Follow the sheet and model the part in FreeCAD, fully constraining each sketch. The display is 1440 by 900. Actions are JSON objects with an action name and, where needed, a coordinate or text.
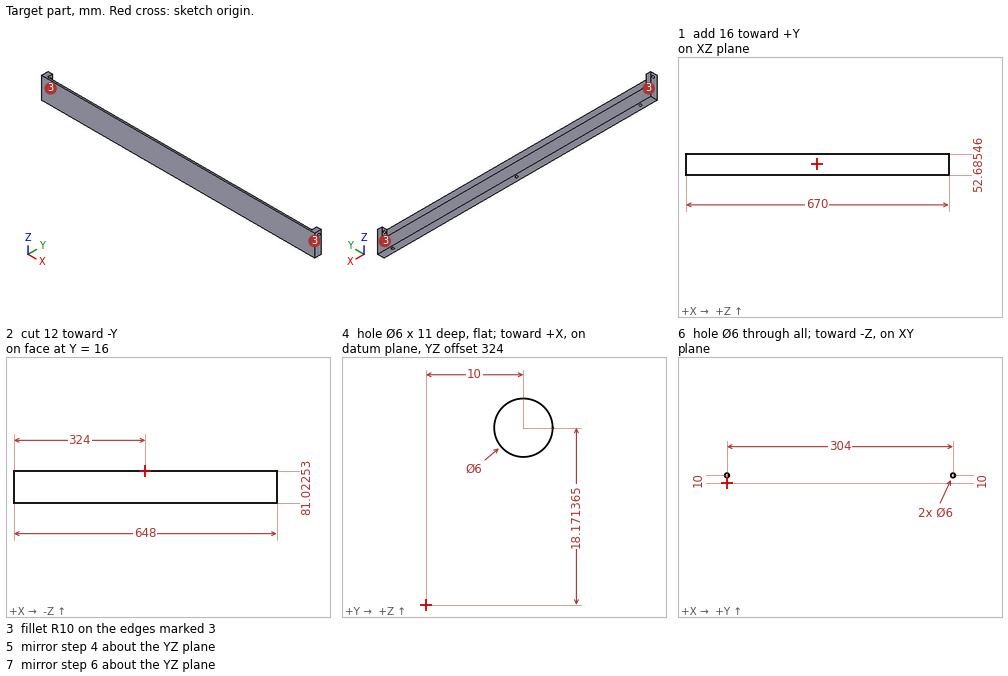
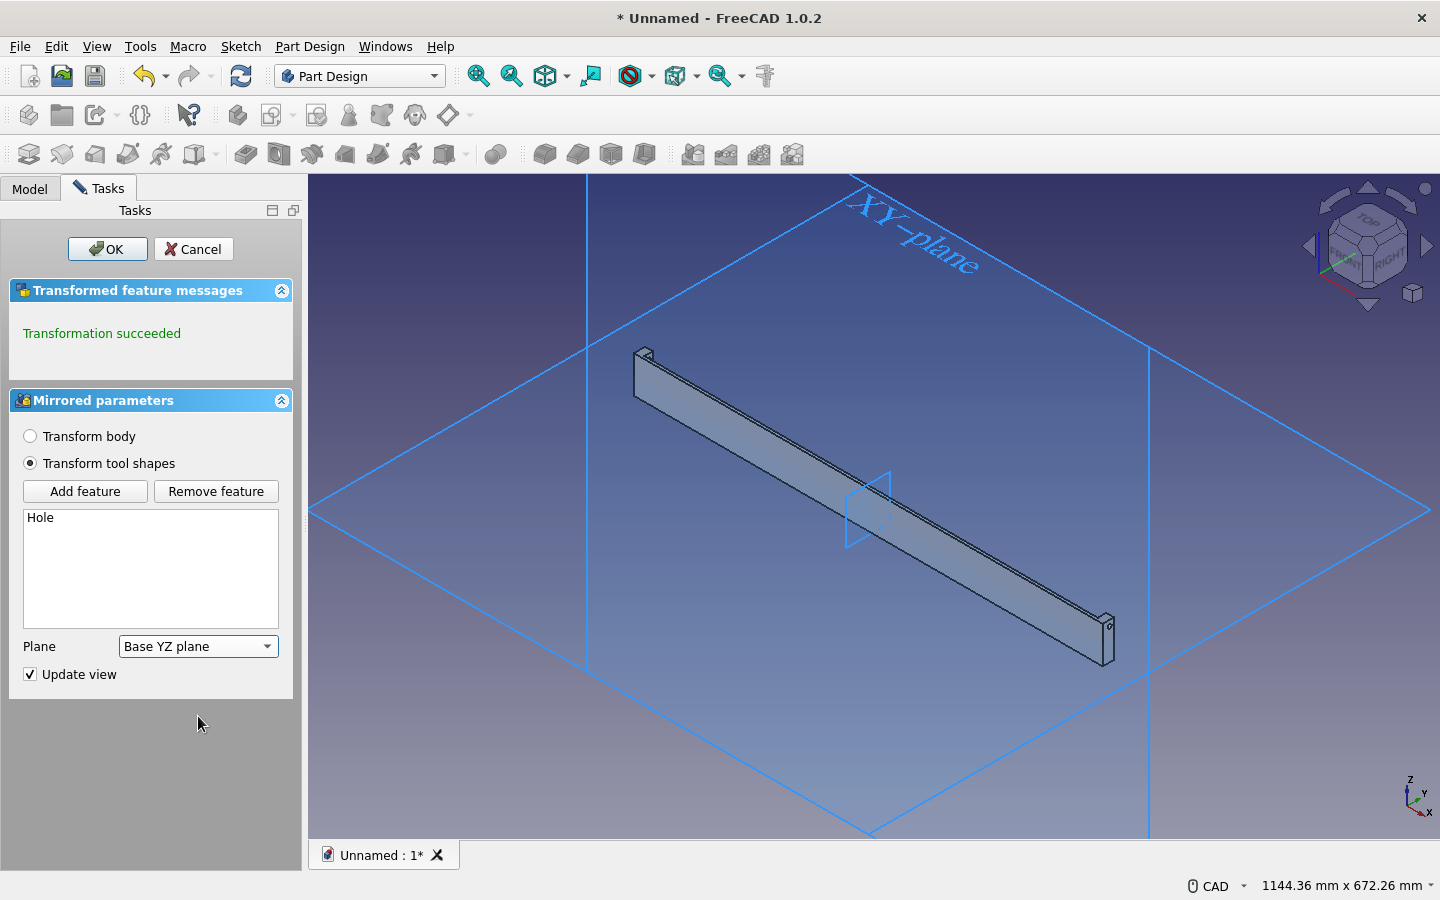
{"action": "left_click", "coordinate": [108, 249]}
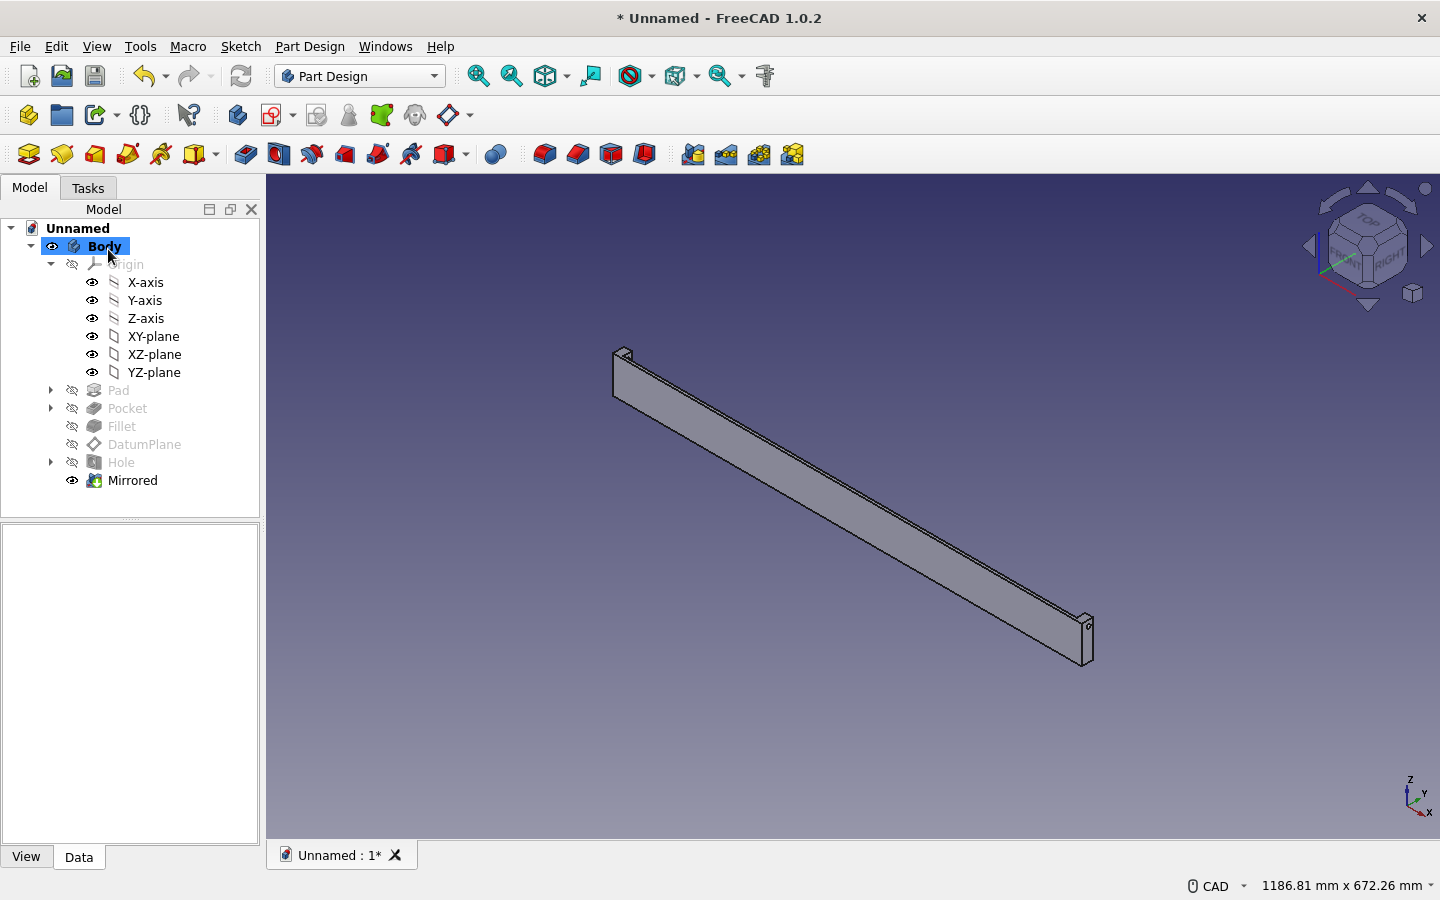
{"action": "left_click", "coordinate": [270, 116]}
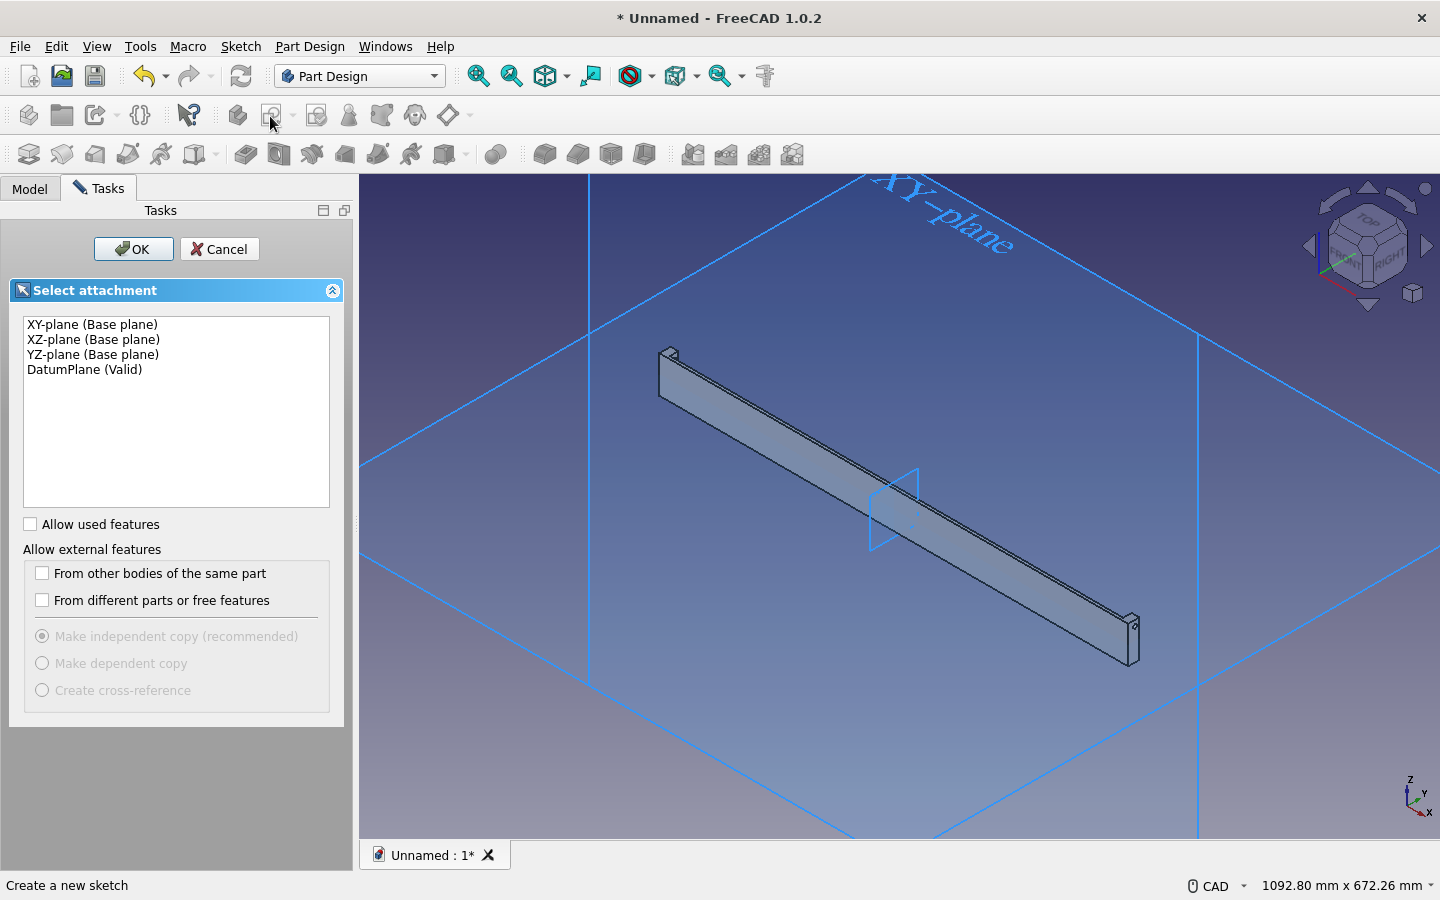
{"action": "left_click", "coordinate": [84, 324]}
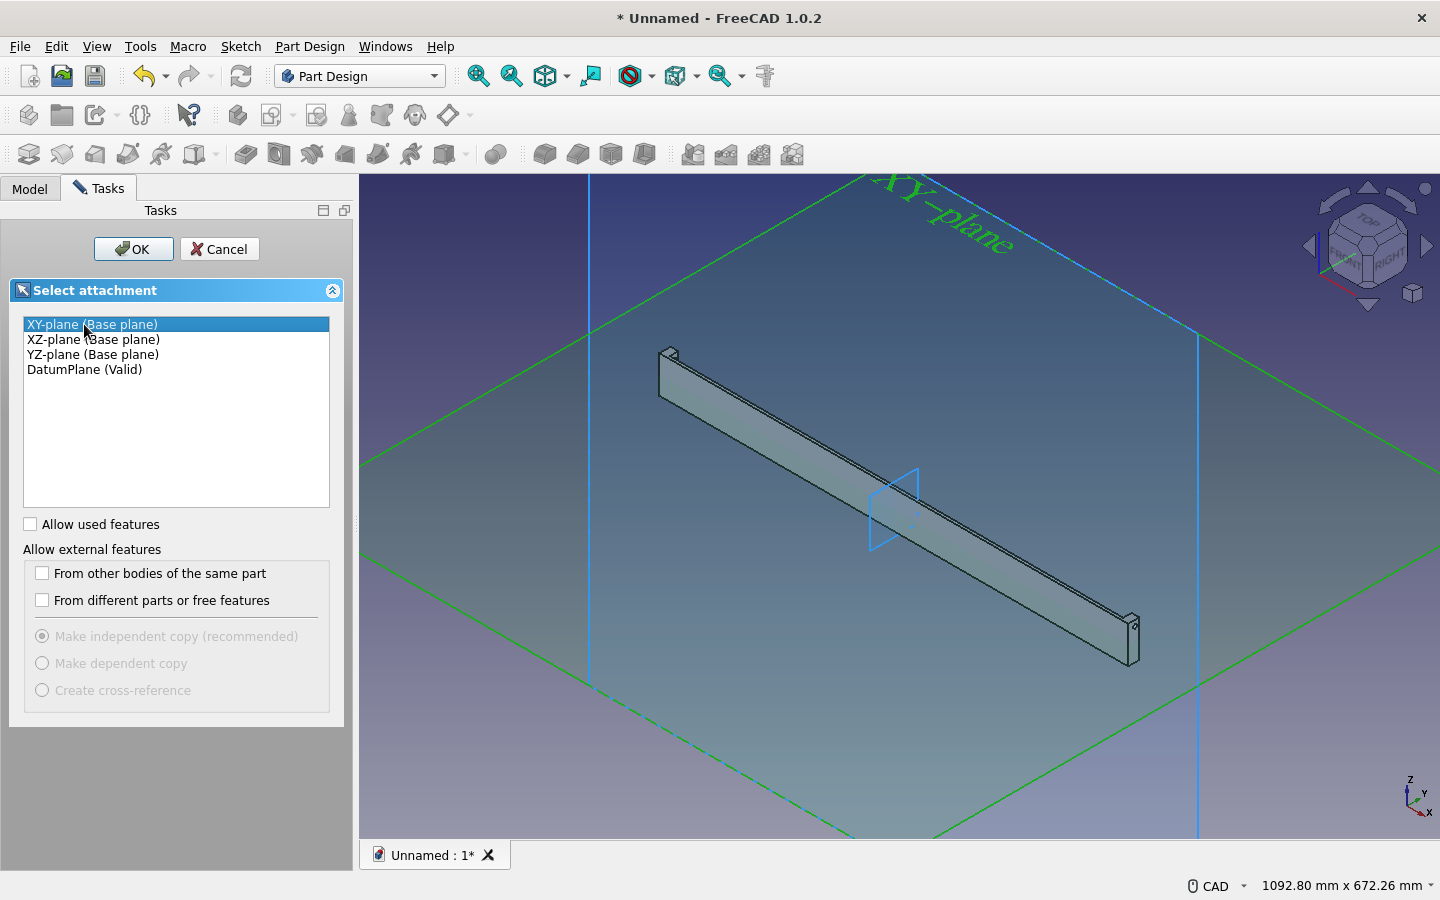
{"action": "left_click", "coordinate": [134, 249]}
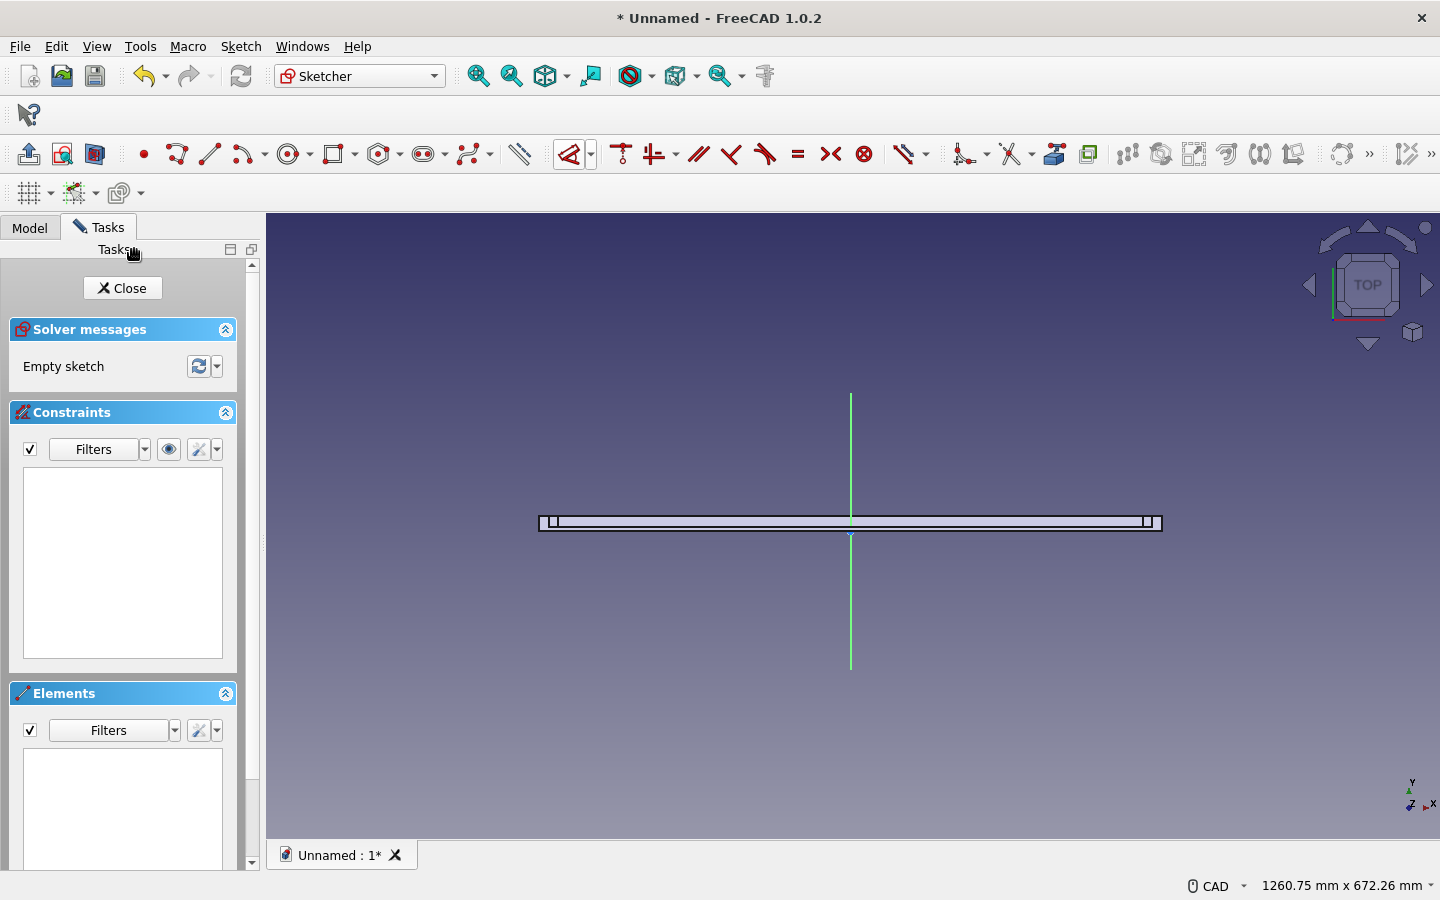
{"action": "left_click", "coordinate": [95, 154]}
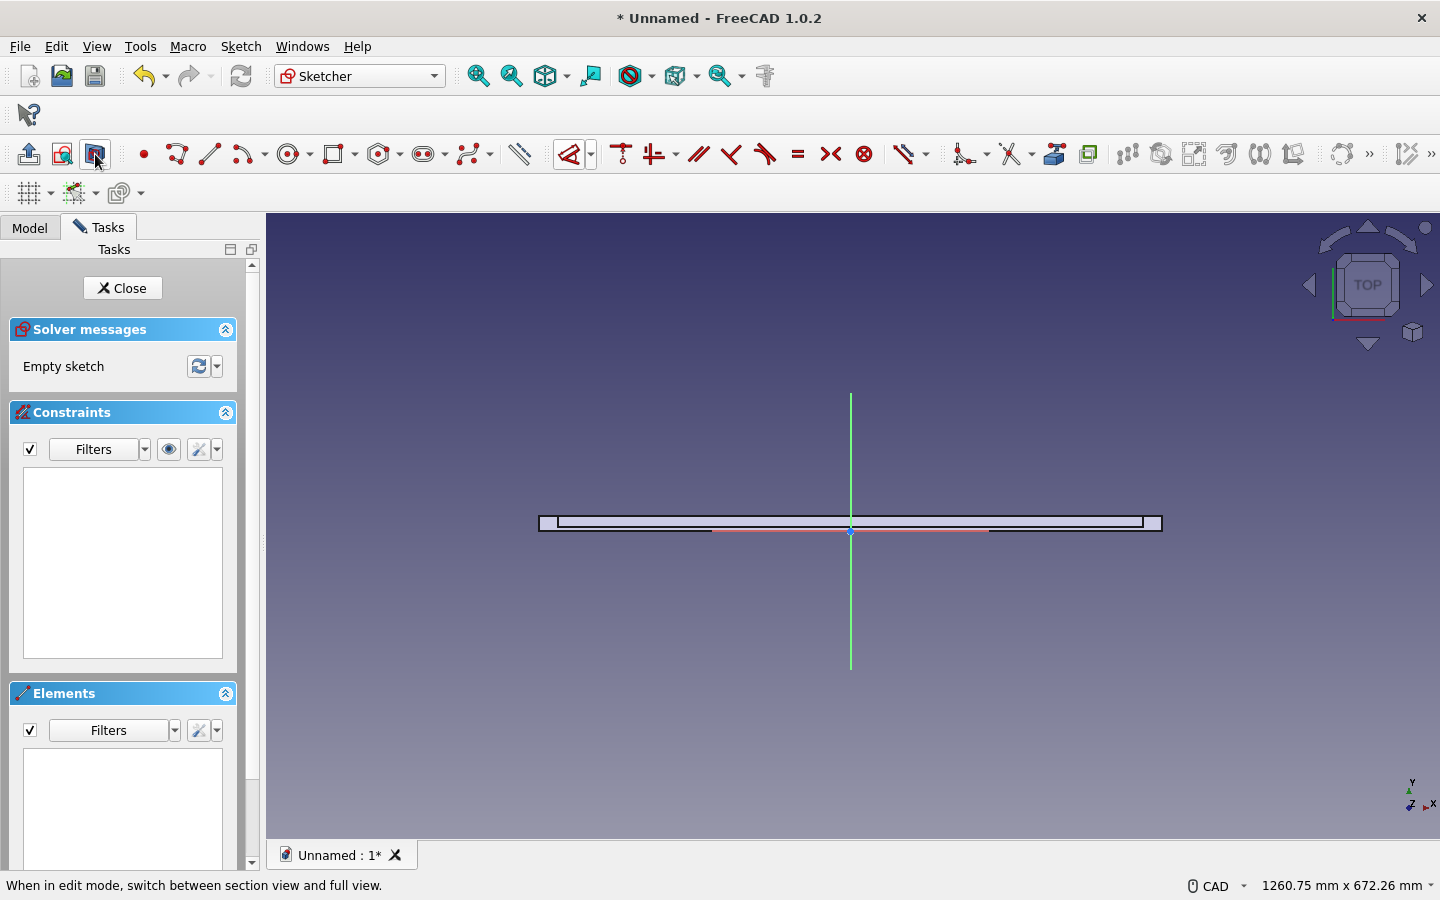
{"action": "scroll", "coordinate": [1161, 524], "scroll_direction": "up", "scroll_amount": 4}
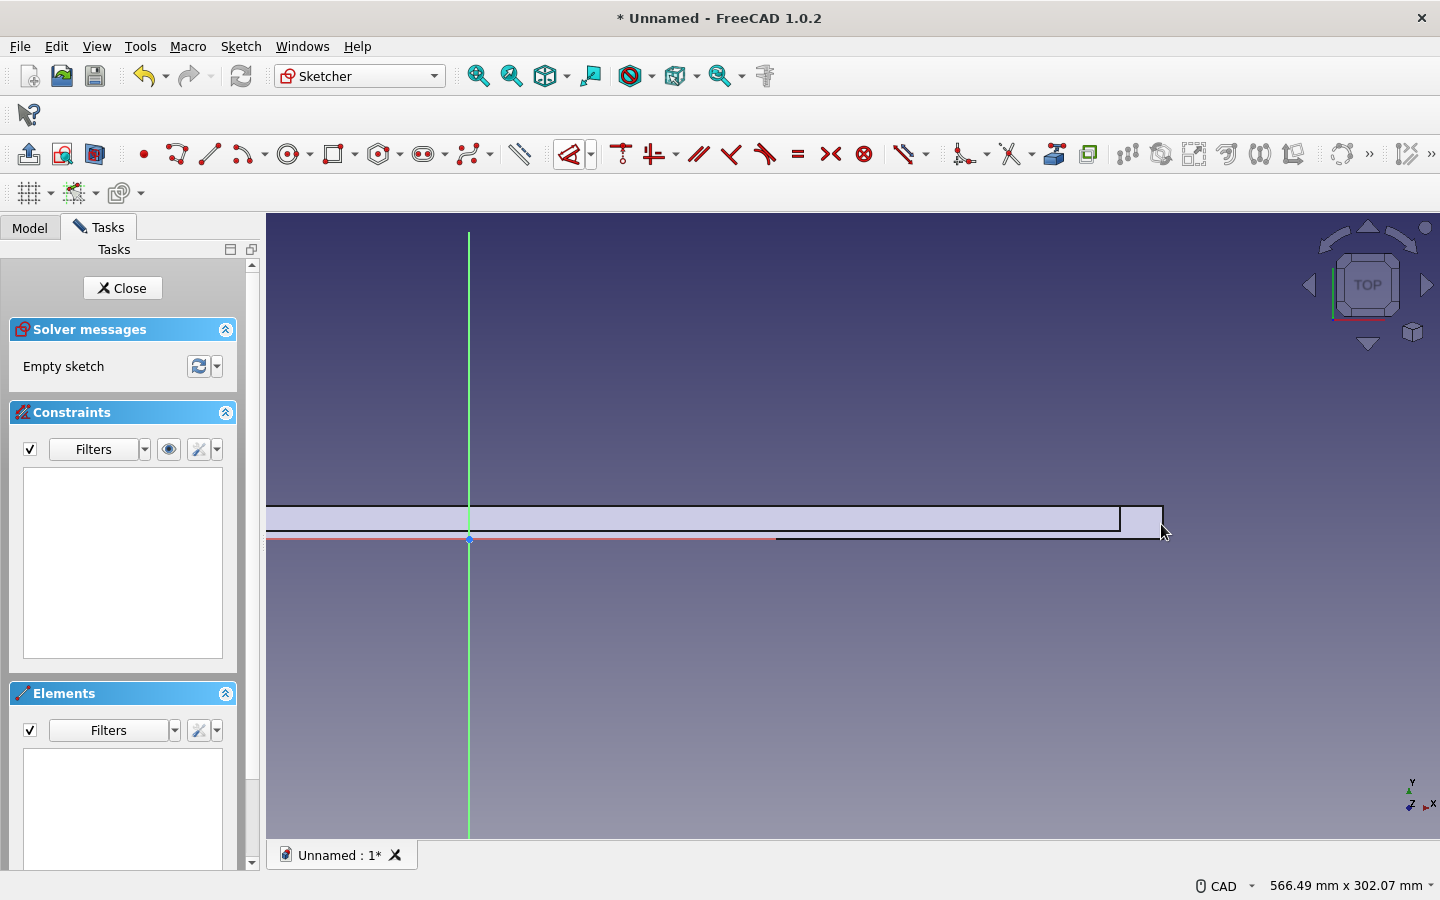
{"action": "left_click", "coordinate": [288, 154]}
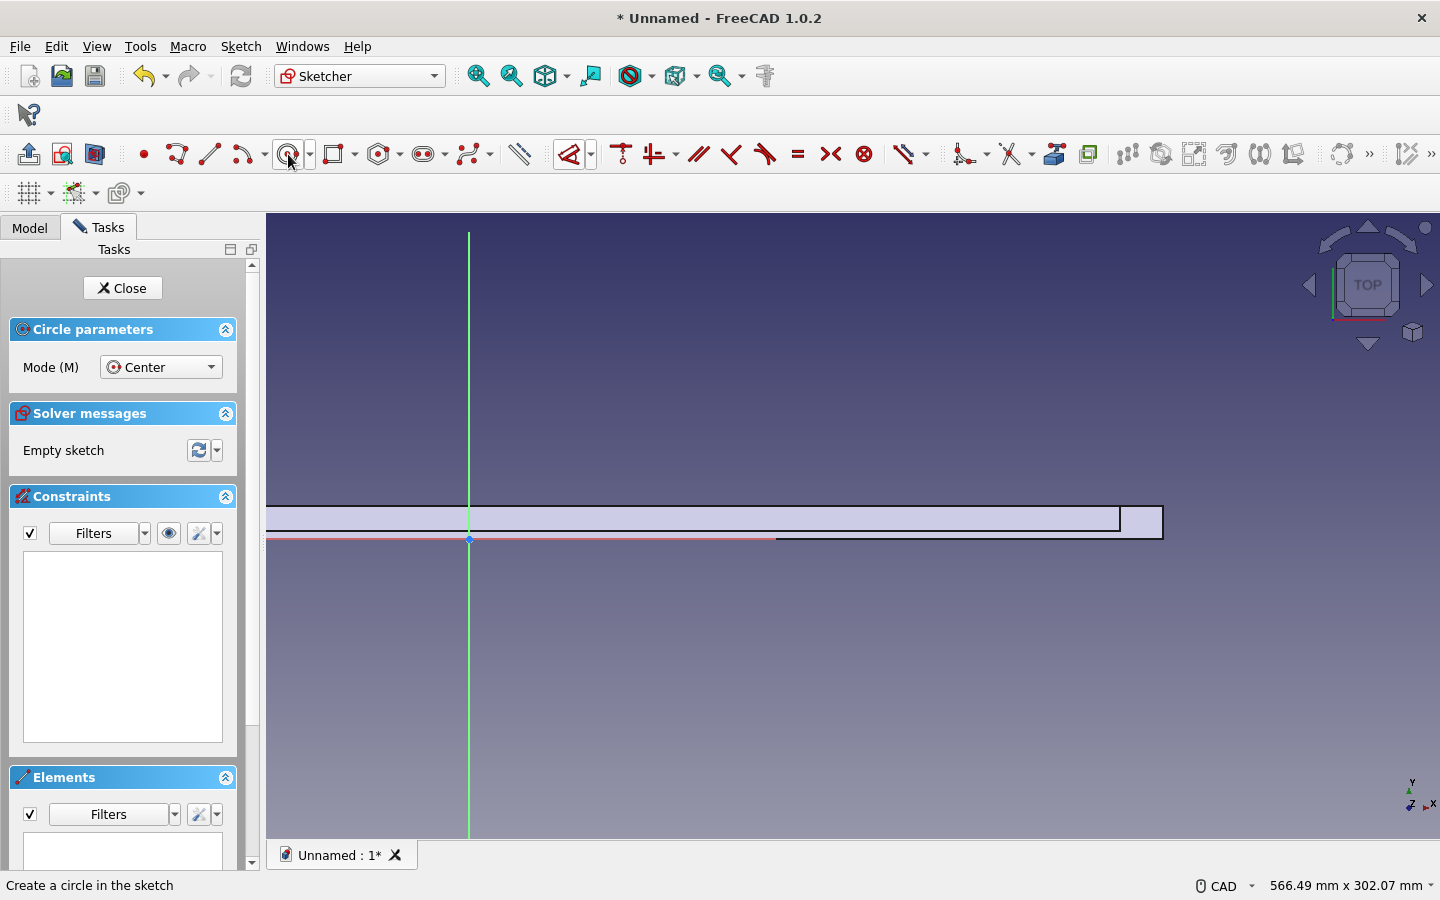
{"action": "scroll", "coordinate": [1099, 518], "scroll_direction": "up", "scroll_amount": 7}